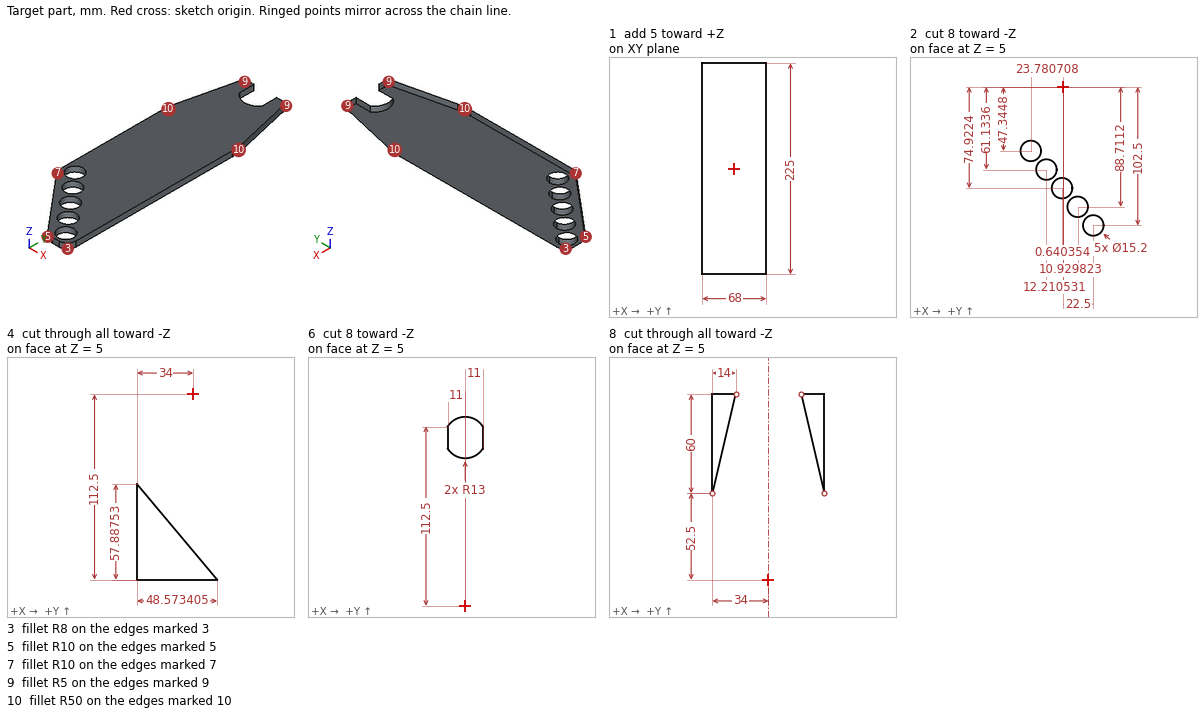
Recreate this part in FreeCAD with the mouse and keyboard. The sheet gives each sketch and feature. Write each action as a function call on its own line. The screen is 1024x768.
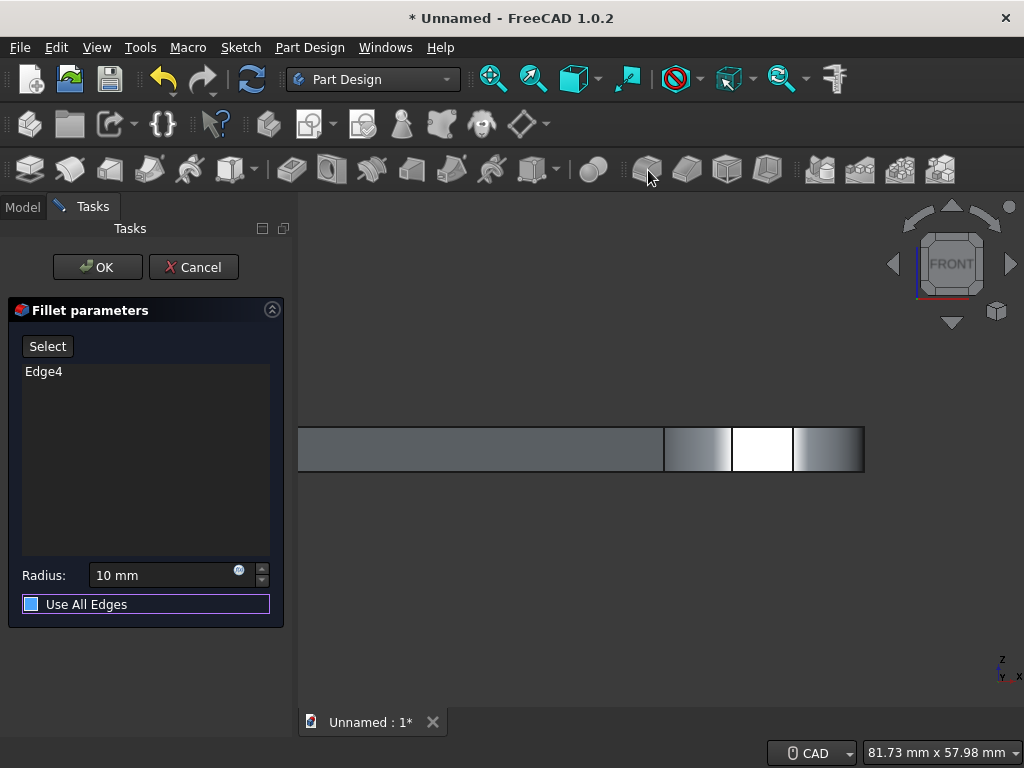
click(98, 267)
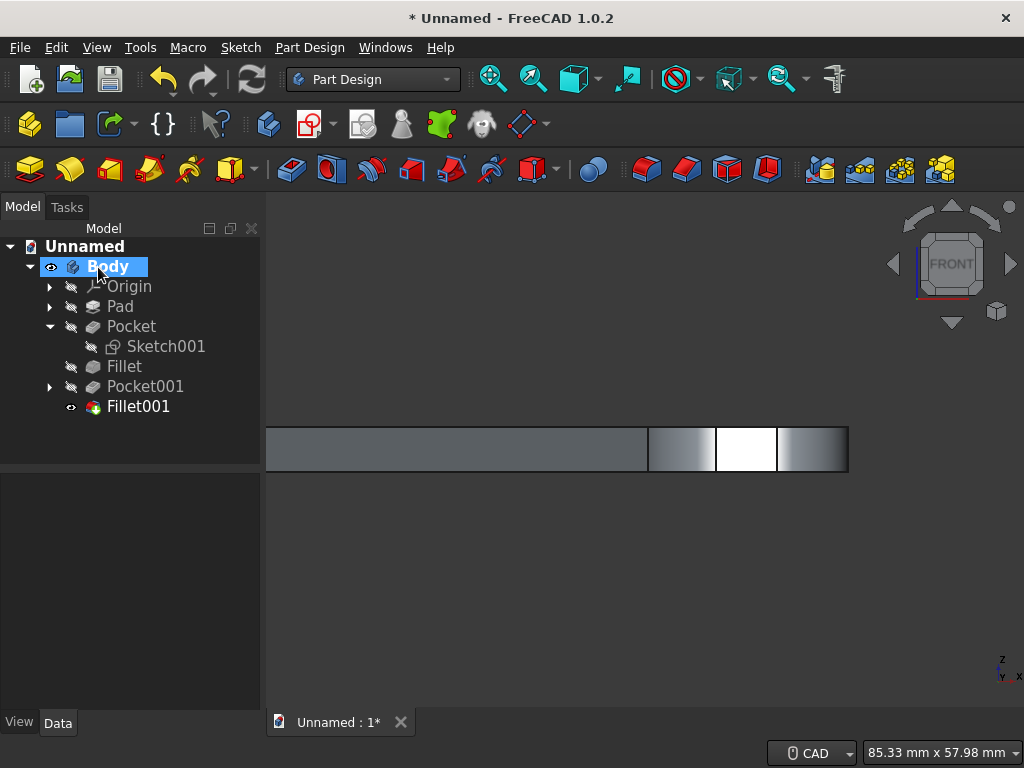
click(494, 80)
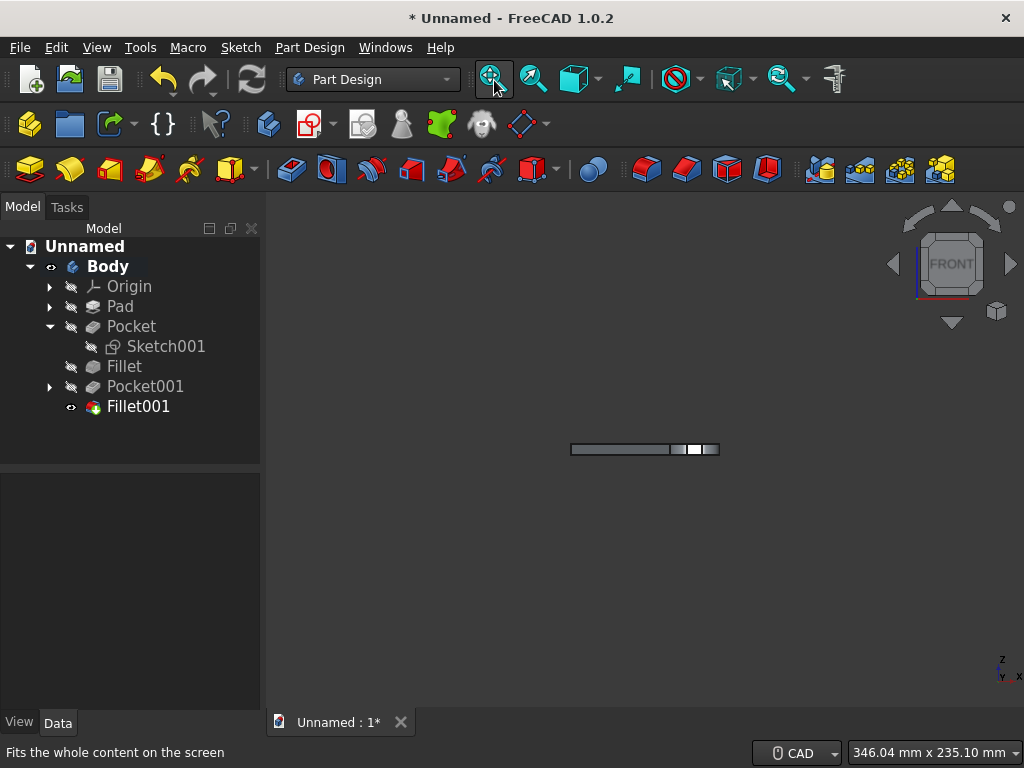
key(0)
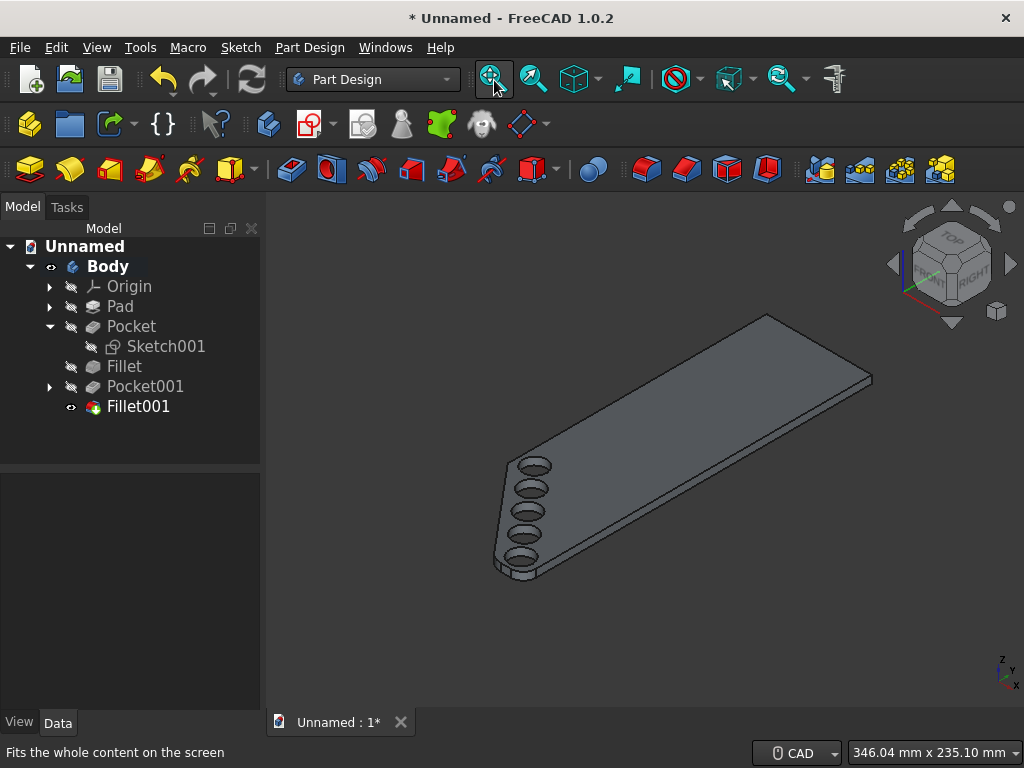
click(745, 387)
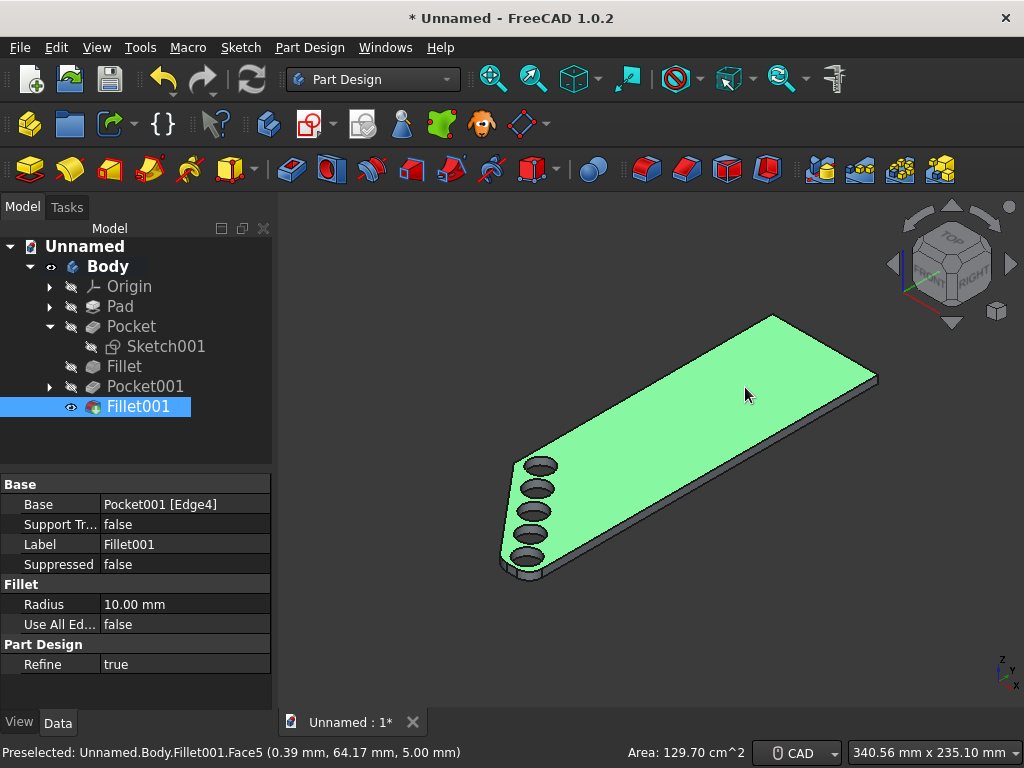
click(310, 124)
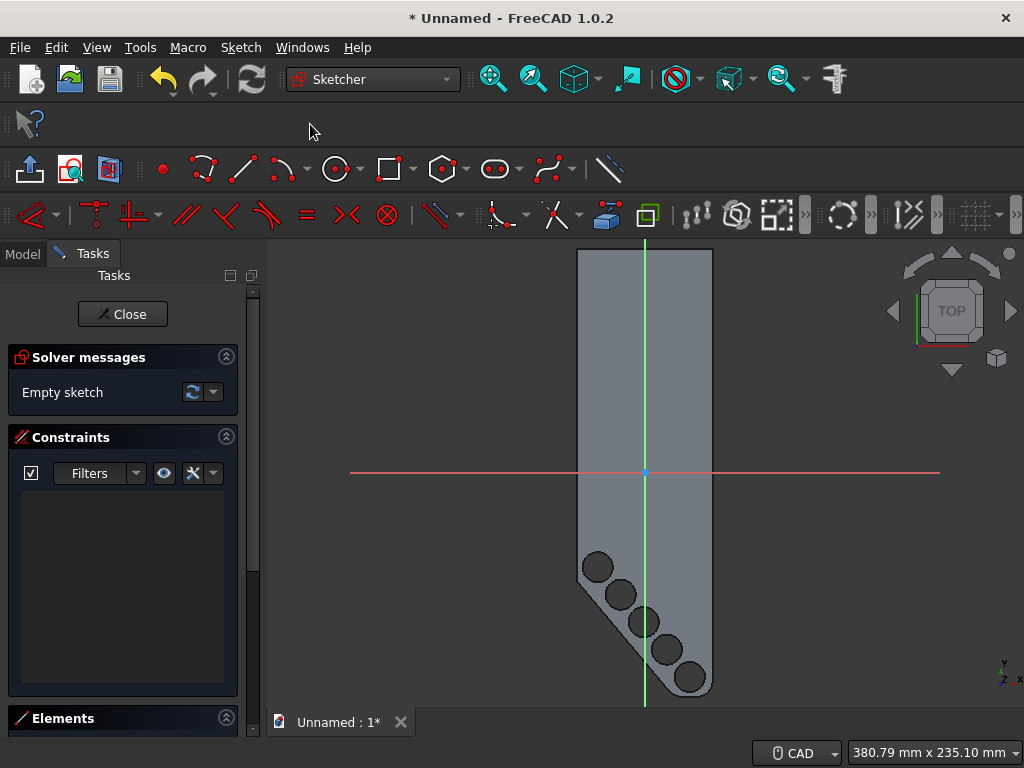
scroll(576, 473, down, 5)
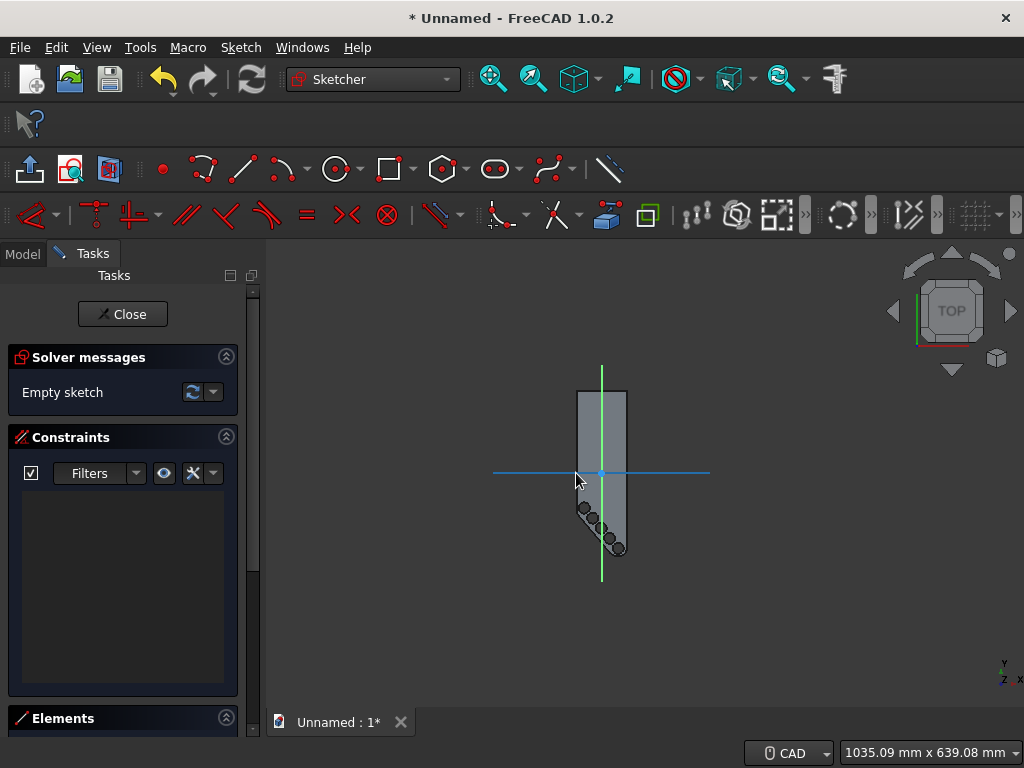
scroll(603, 391, up, 14)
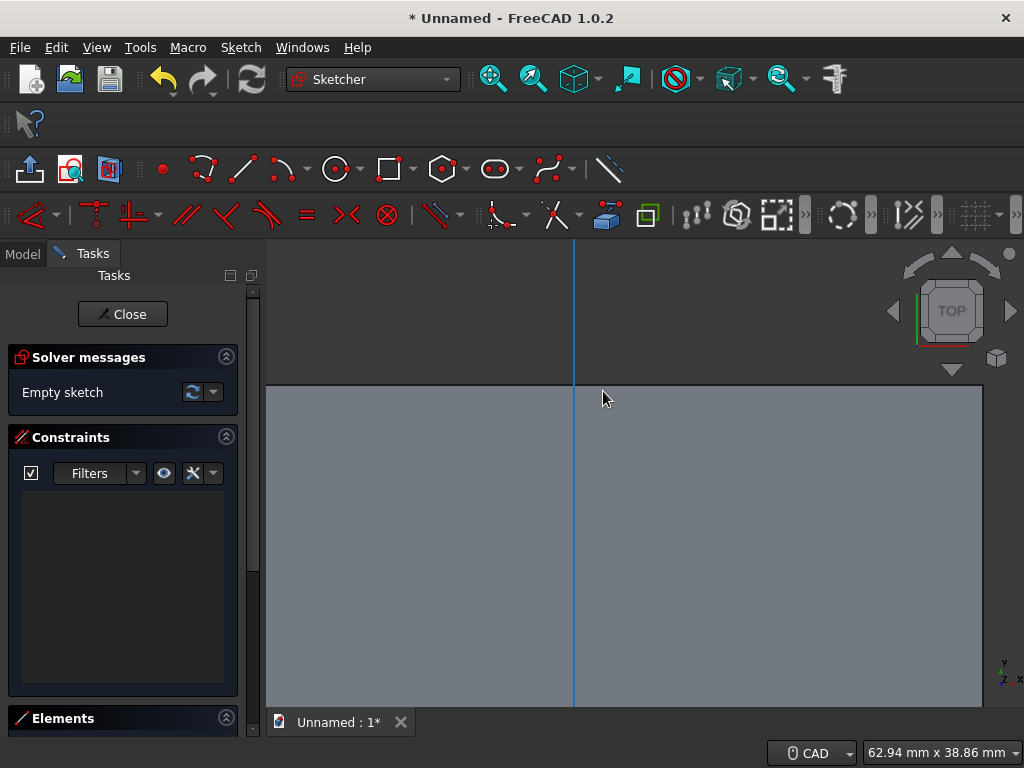
click(244, 170)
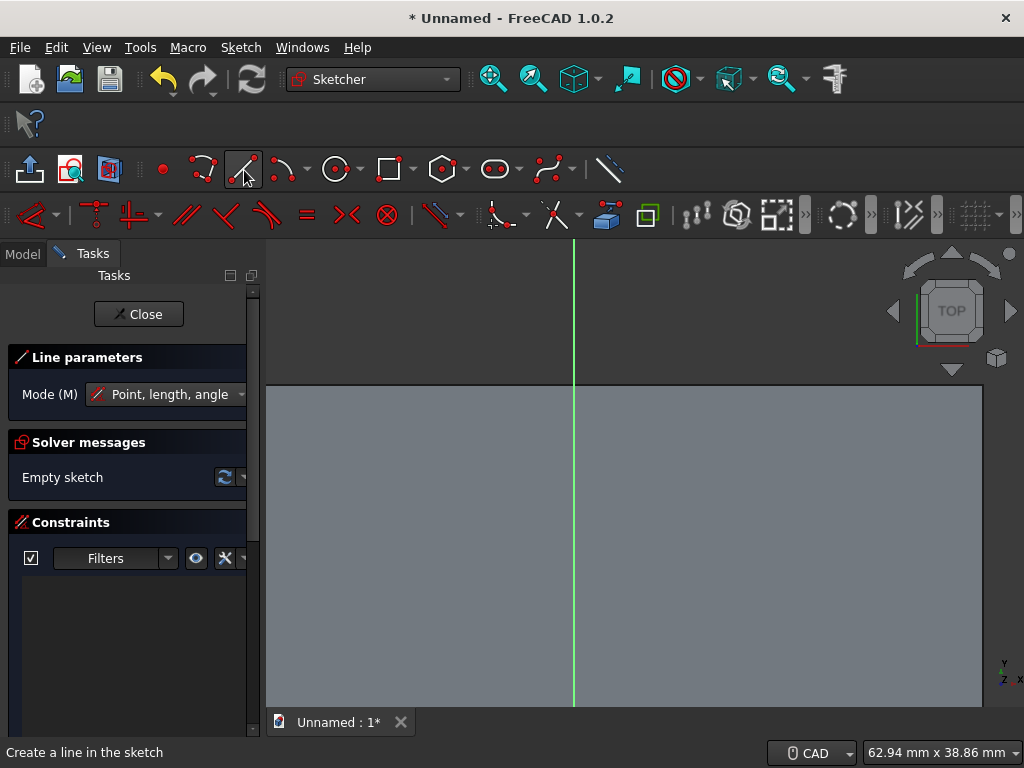
click(441, 385)
click(441, 552)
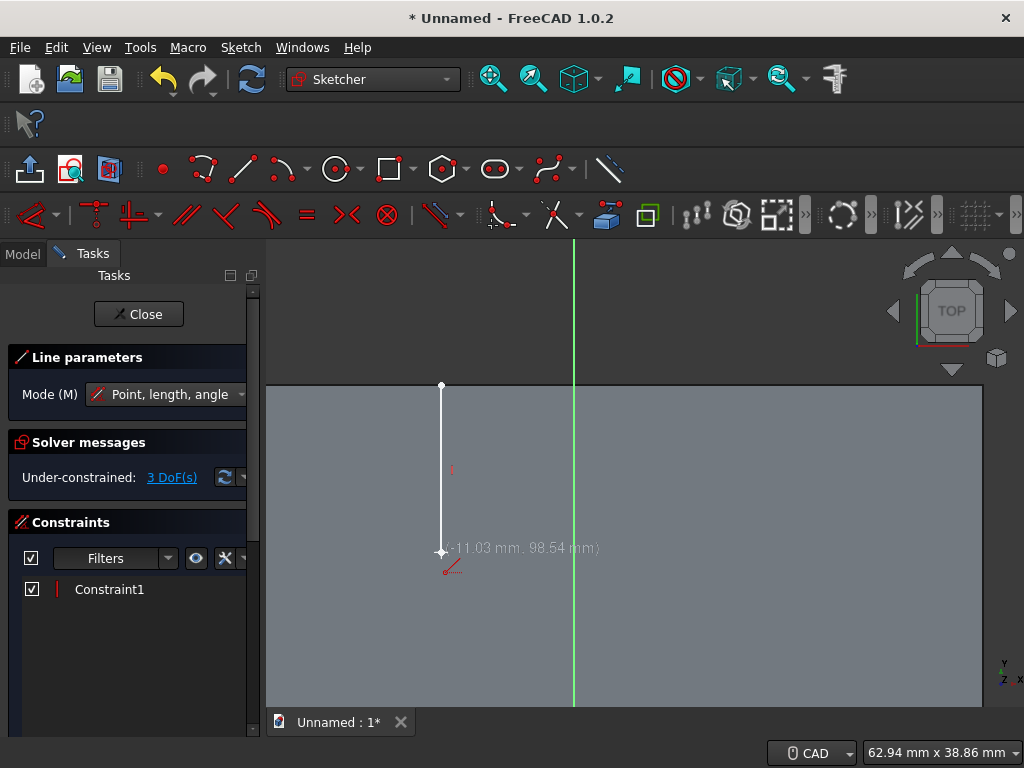
click(706, 552)
click(706, 385)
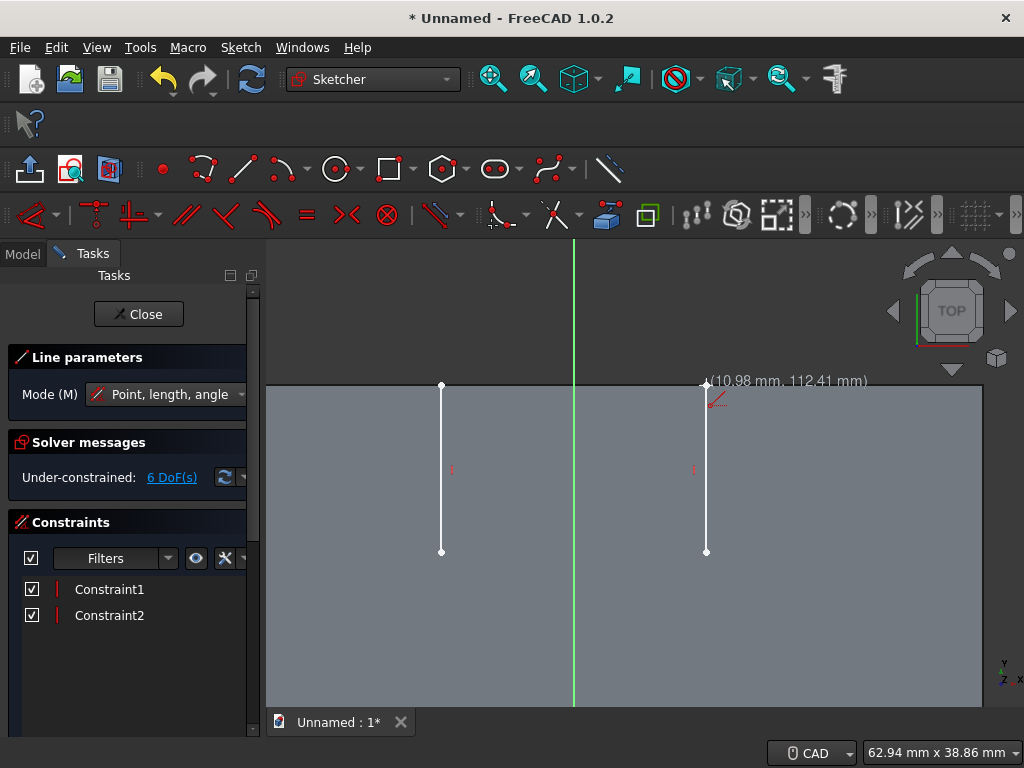
key(g)
key(3)
key(a)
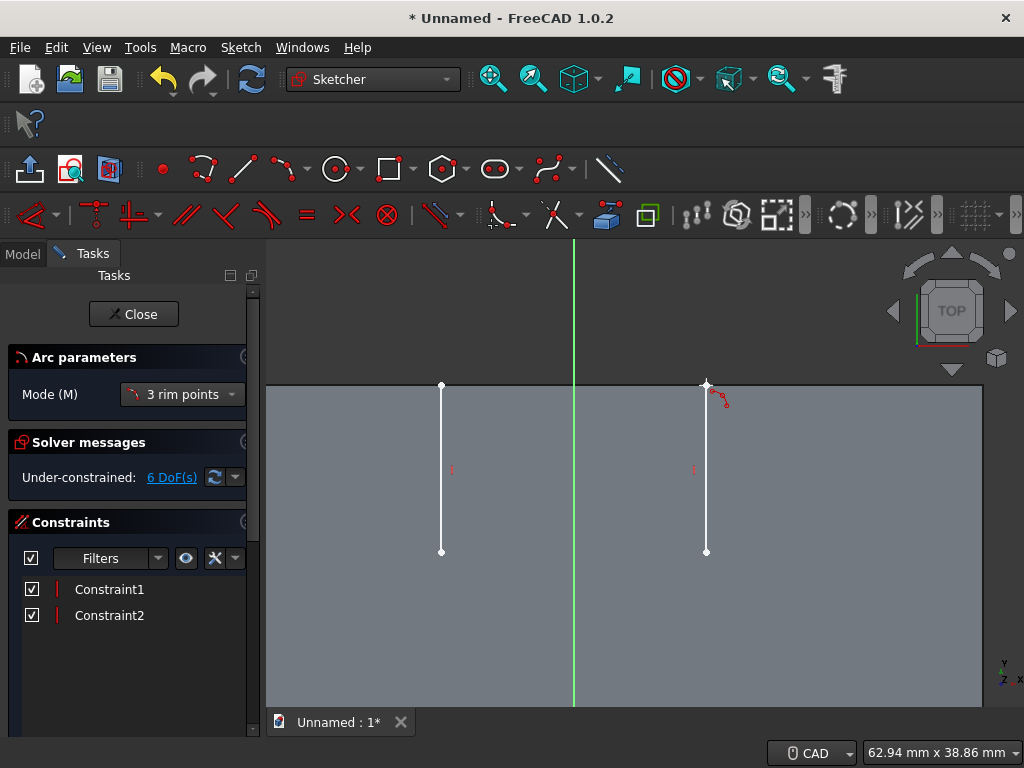
click(441, 553)
click(706, 553)
click(542, 622)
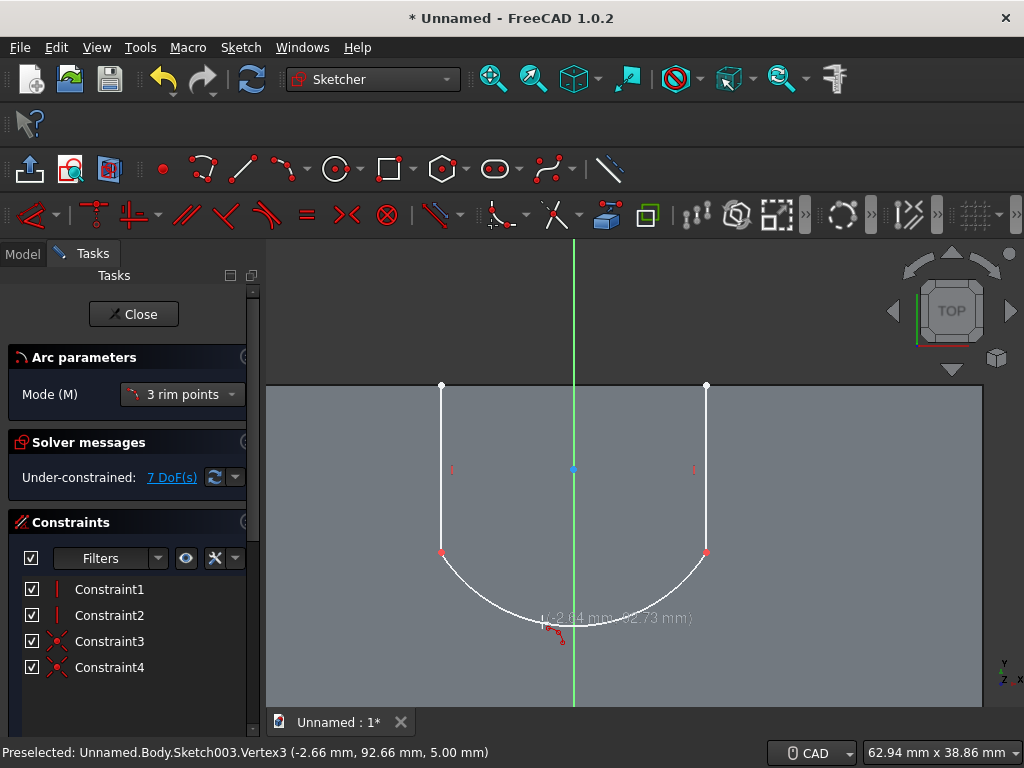
click(706, 386)
click(441, 386)
click(605, 315)
key(Escape)